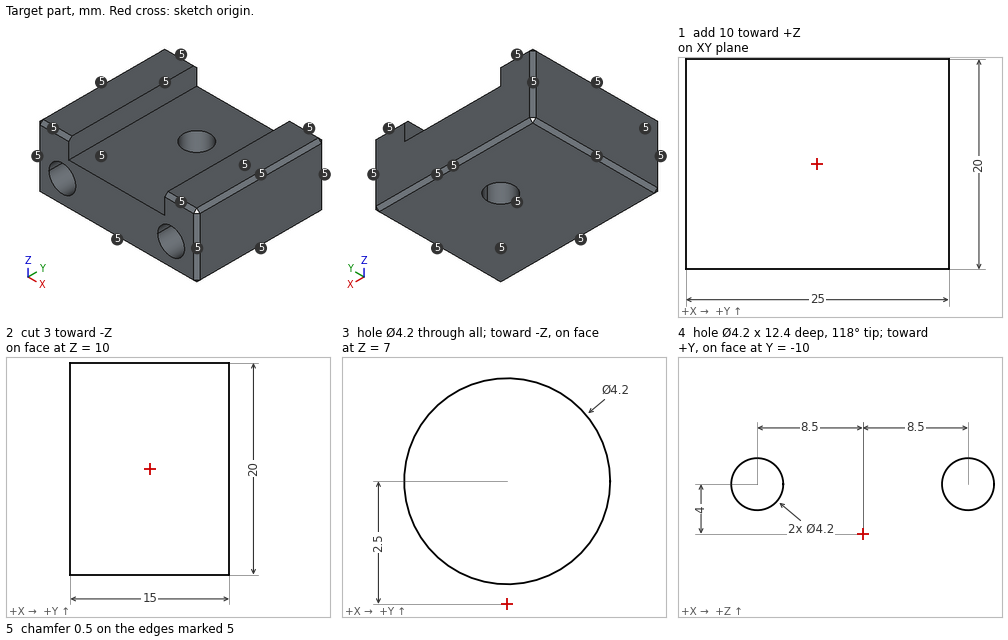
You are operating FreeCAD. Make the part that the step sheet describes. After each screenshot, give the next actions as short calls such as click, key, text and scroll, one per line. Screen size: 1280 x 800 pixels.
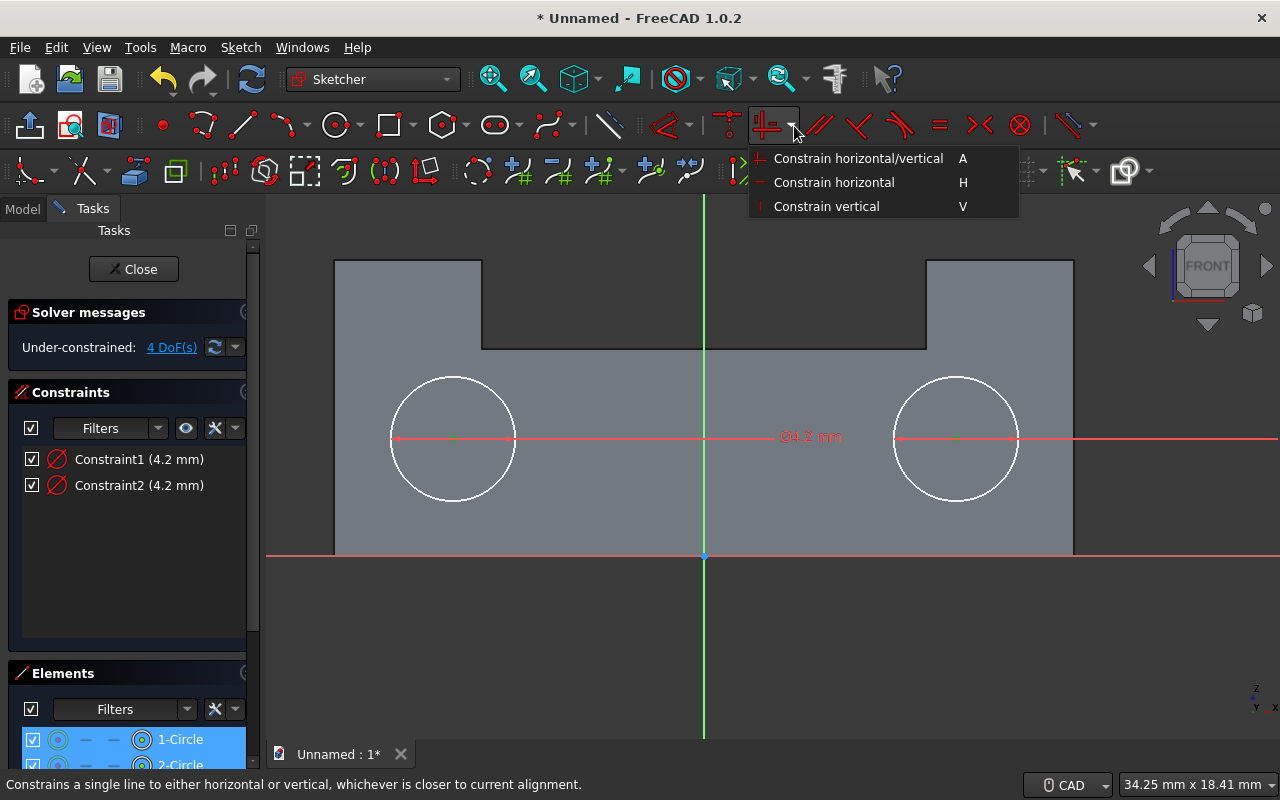
click(884, 182)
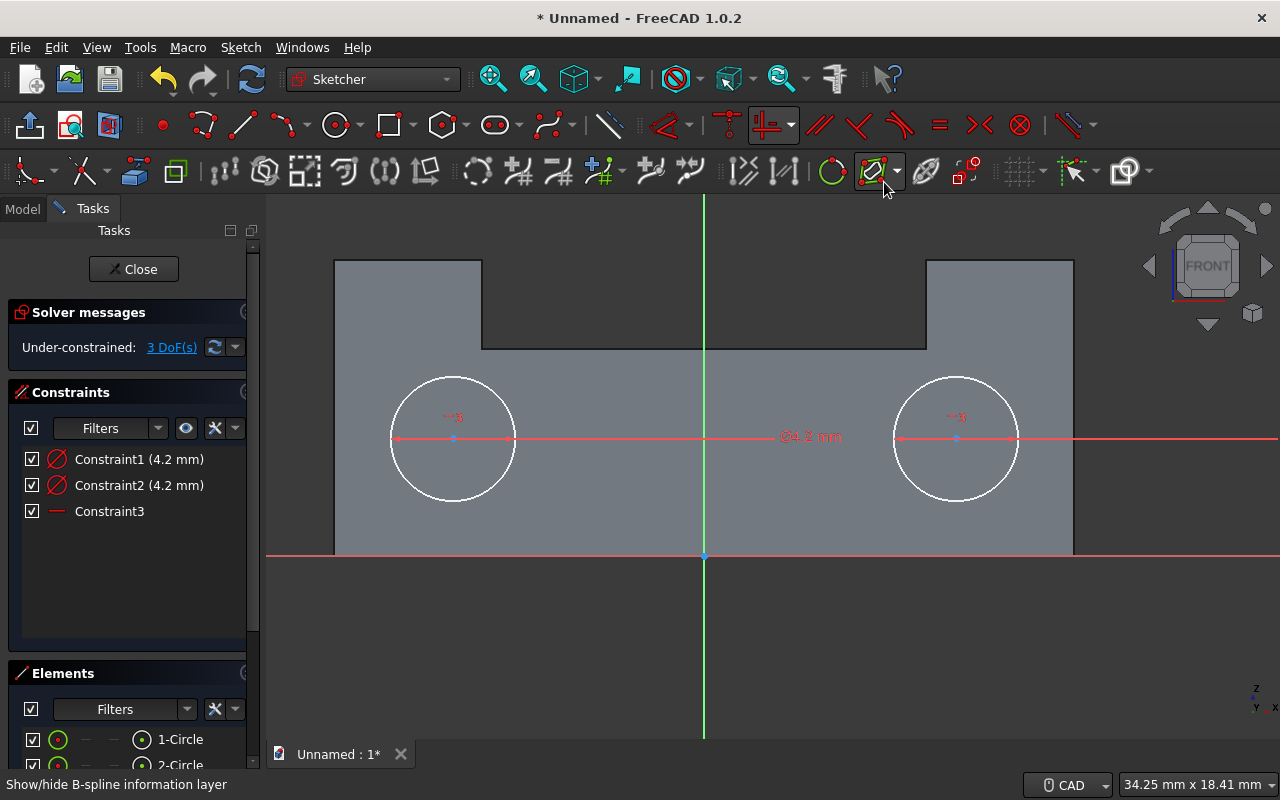
click(664, 126)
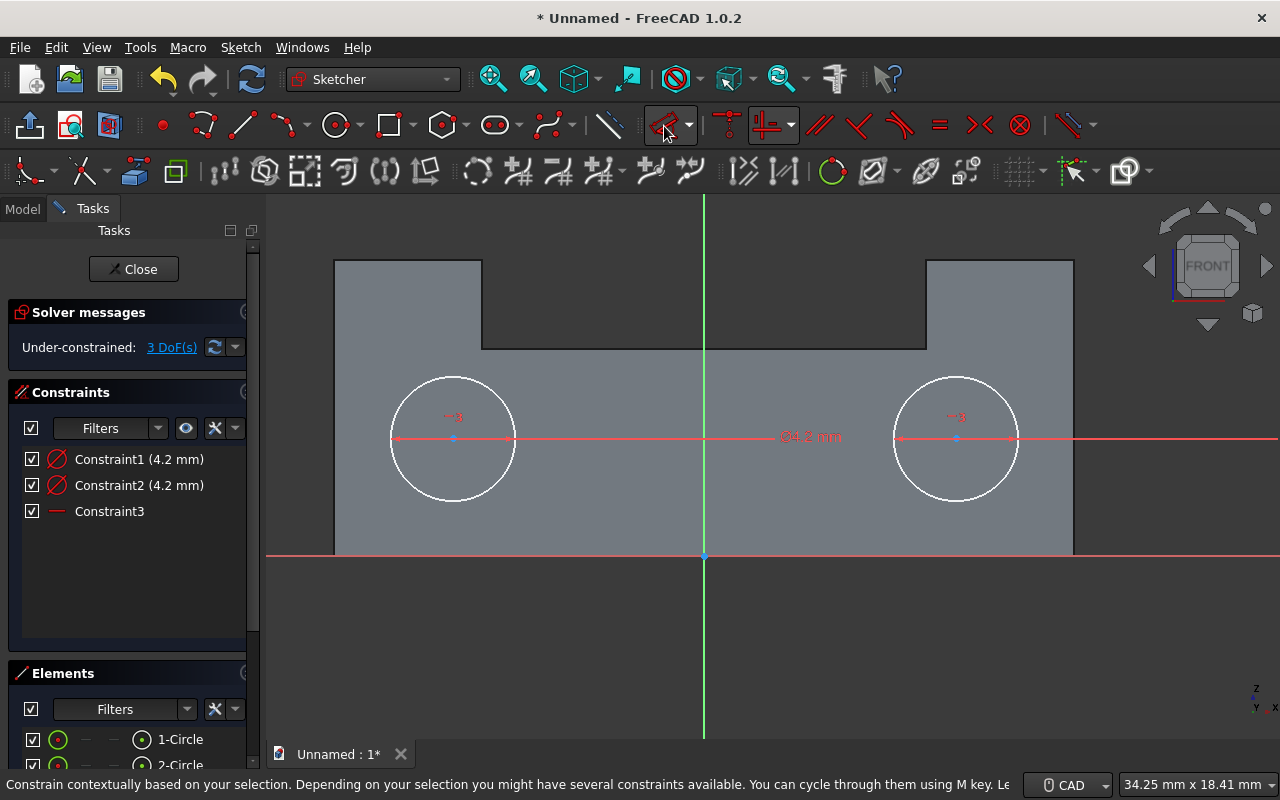
click(453, 439)
click(419, 471)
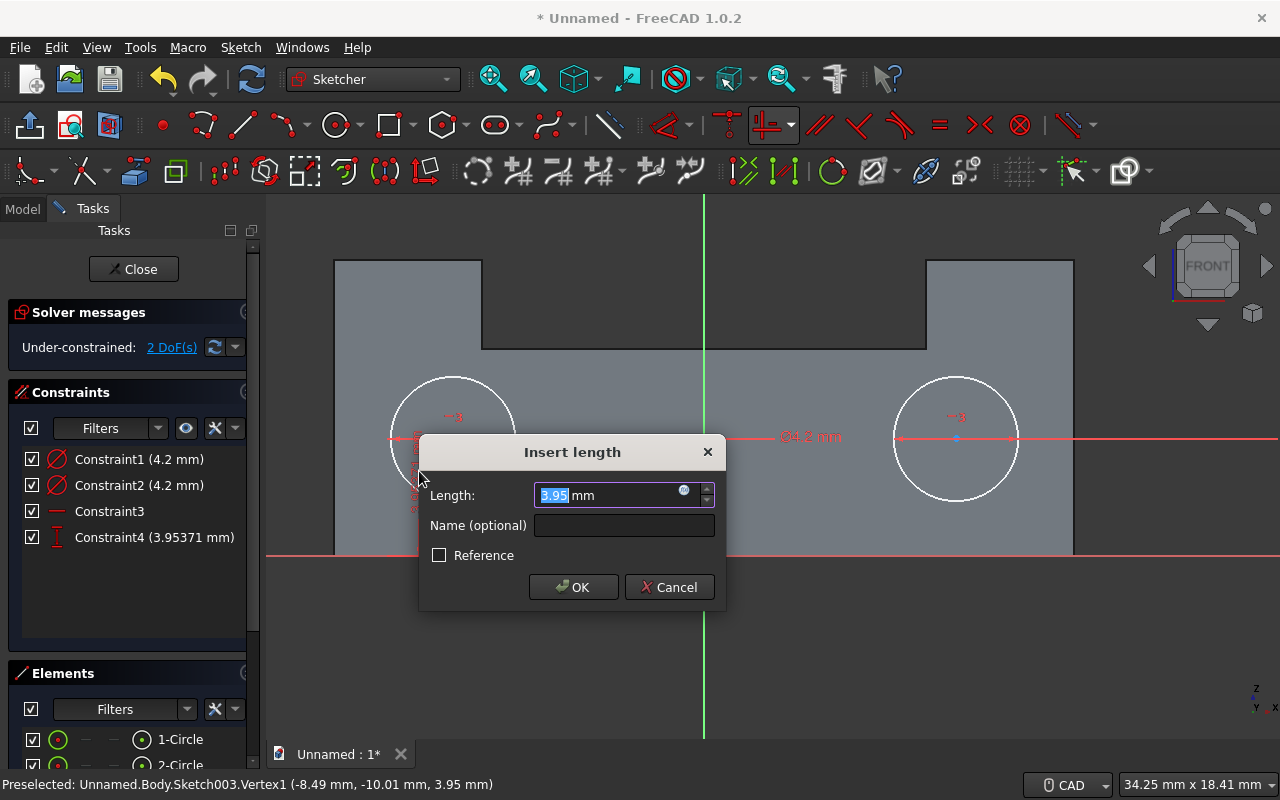
text(4)
key(Return)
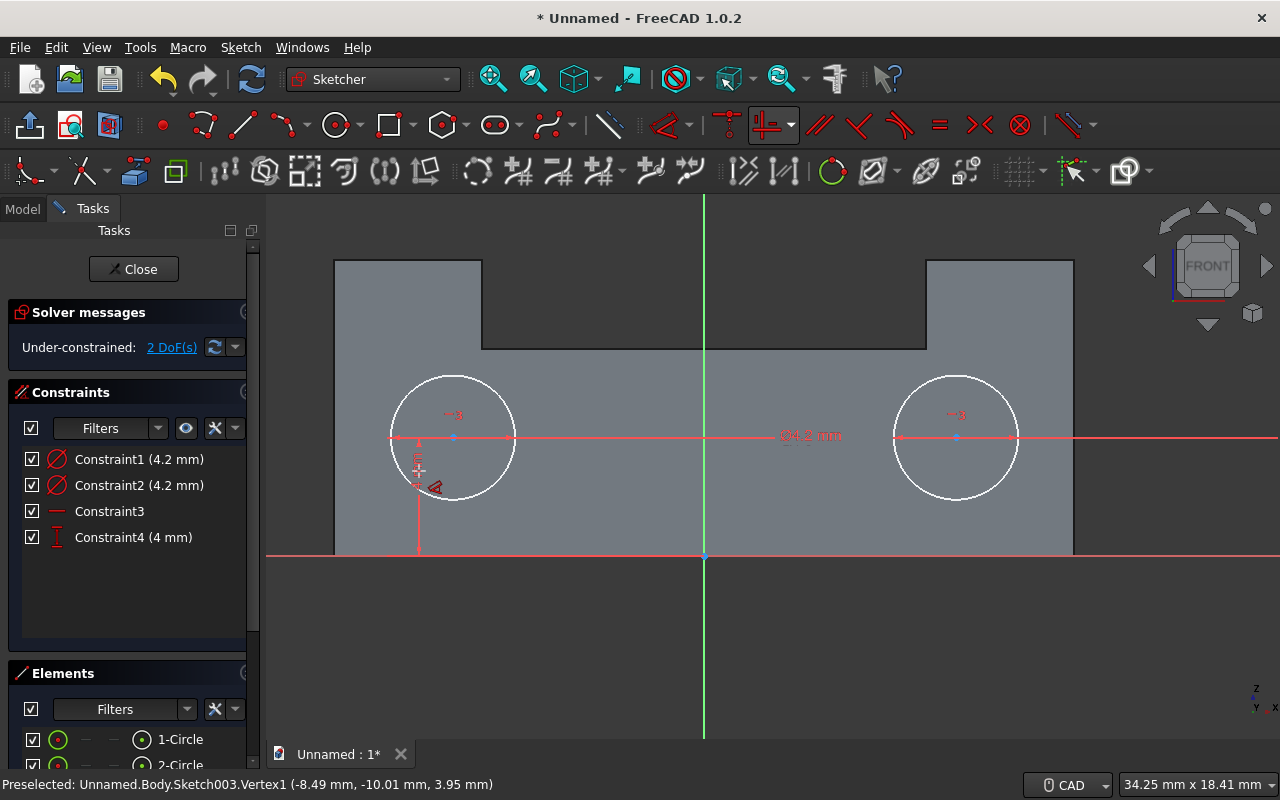
click(453, 438)
click(579, 590)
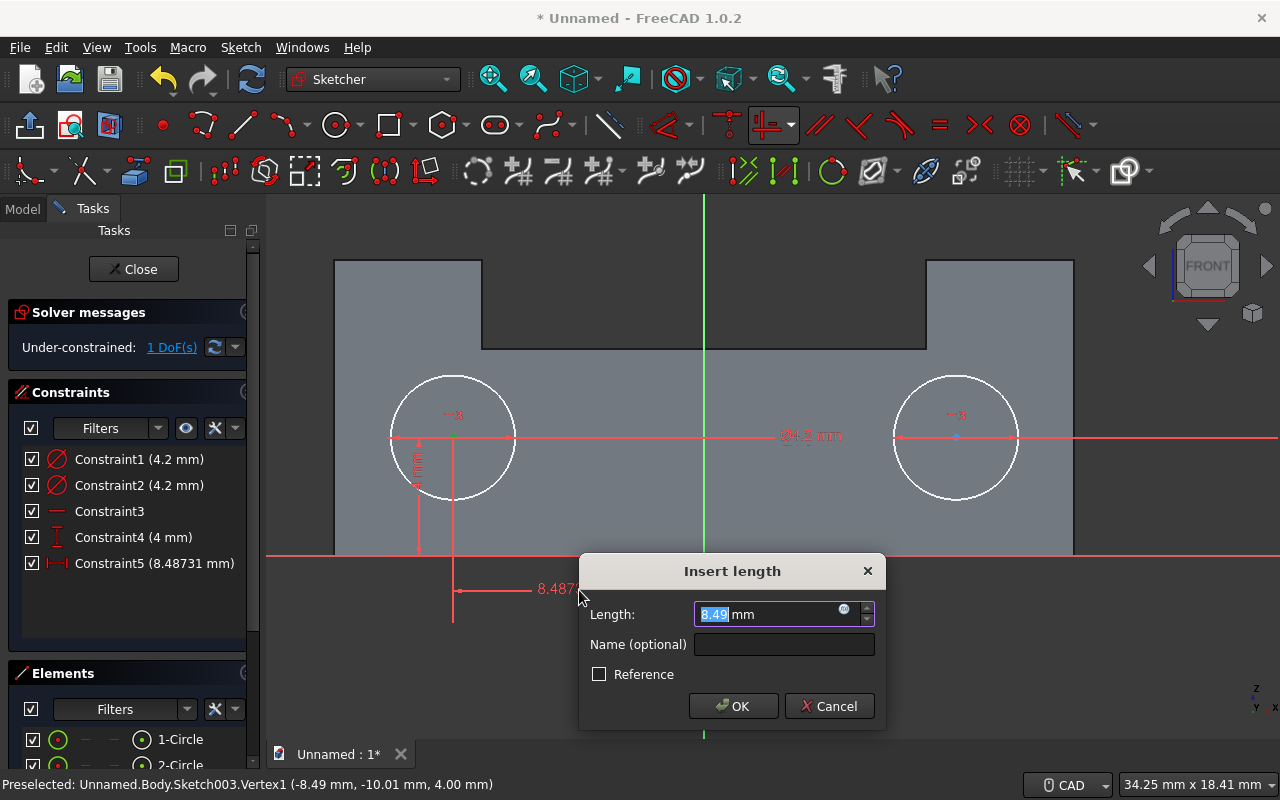
text(8.5)
key(Return)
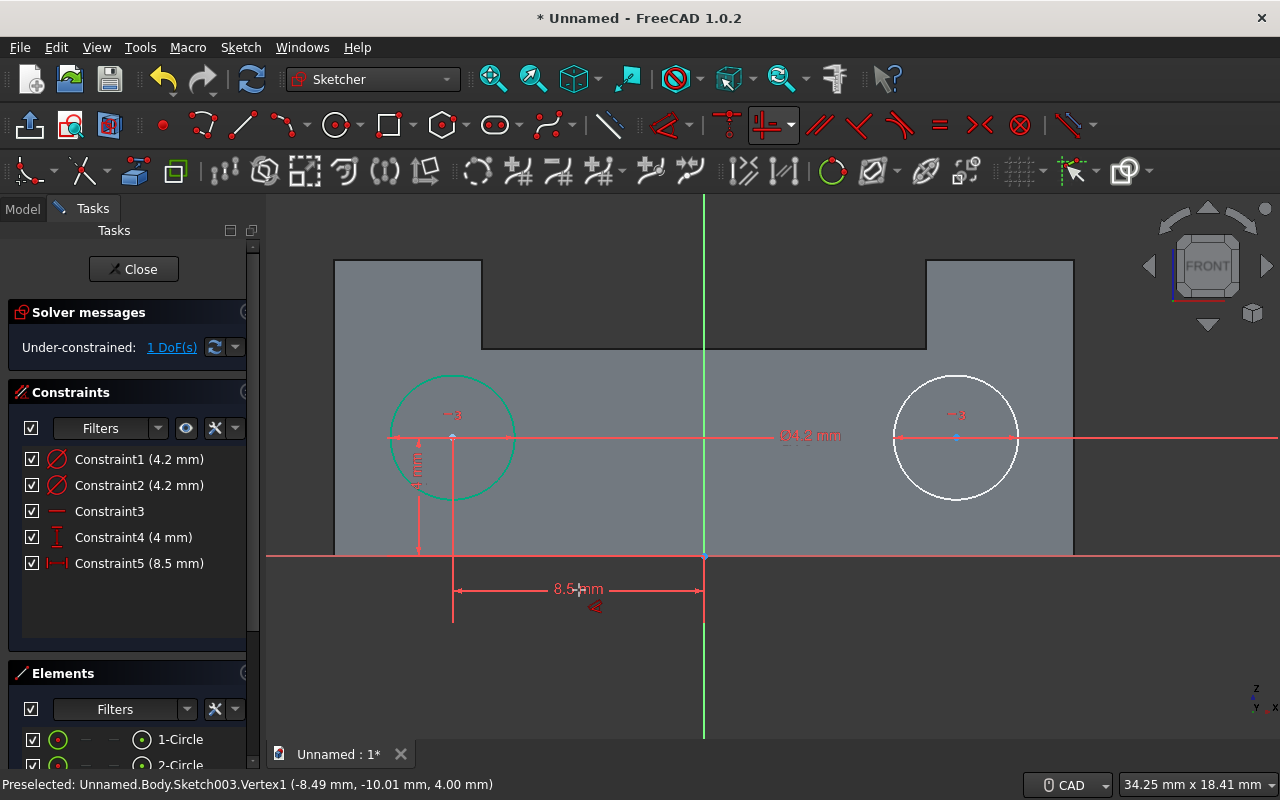
click(956, 438)
click(830, 590)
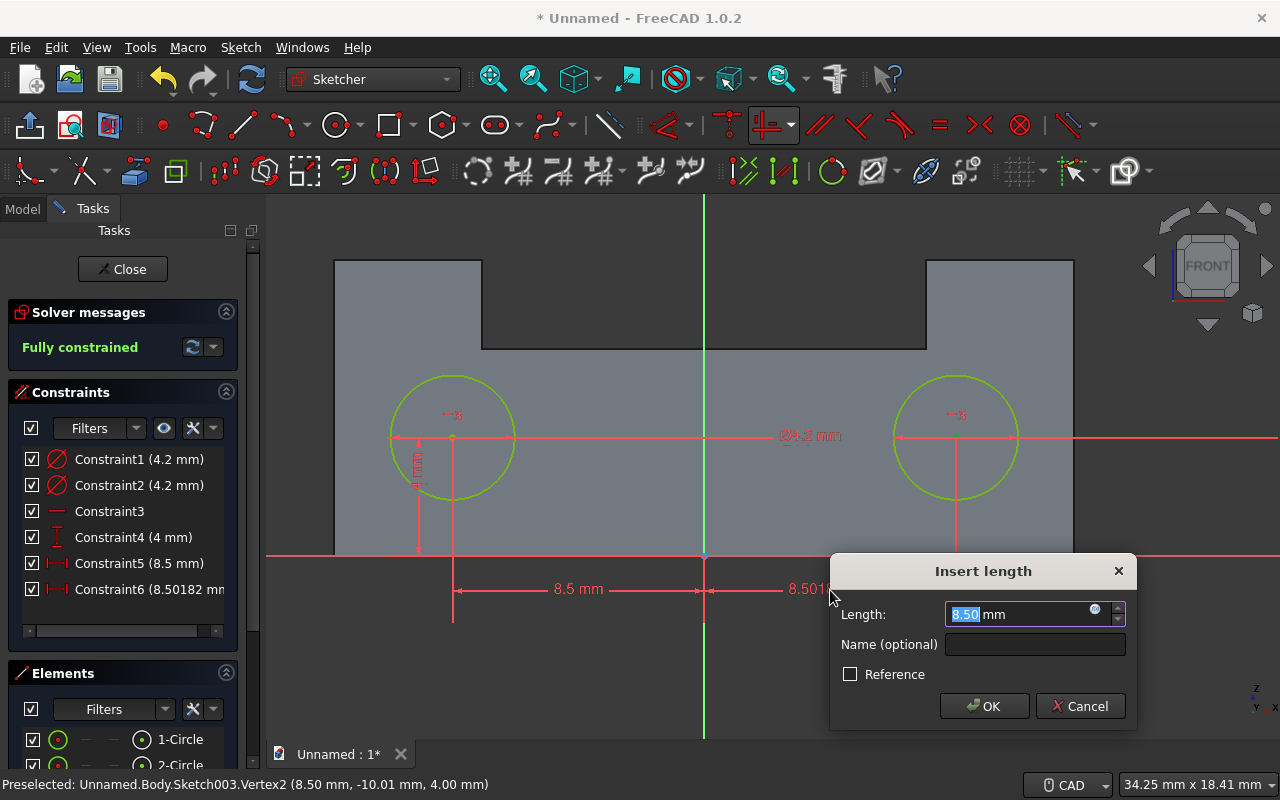
text(8.5)
key(Return)
key(Escape)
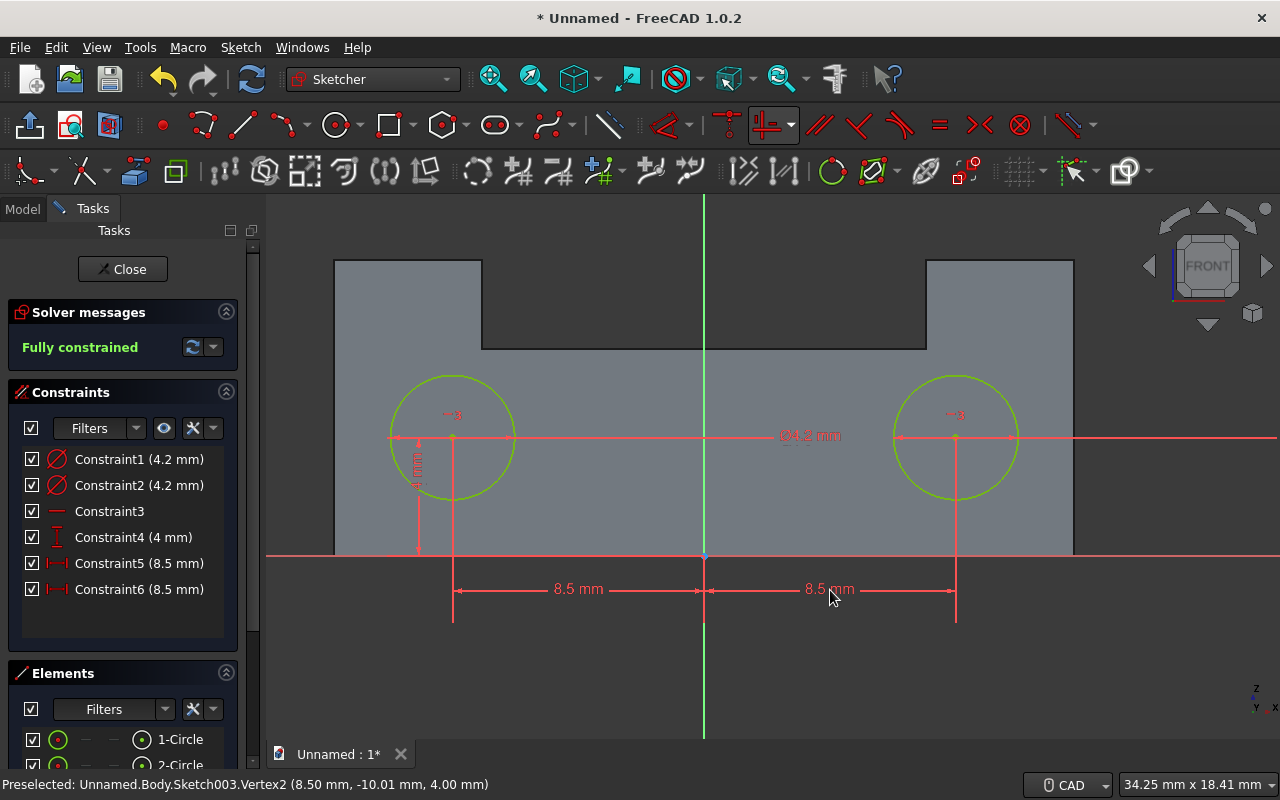
click(123, 269)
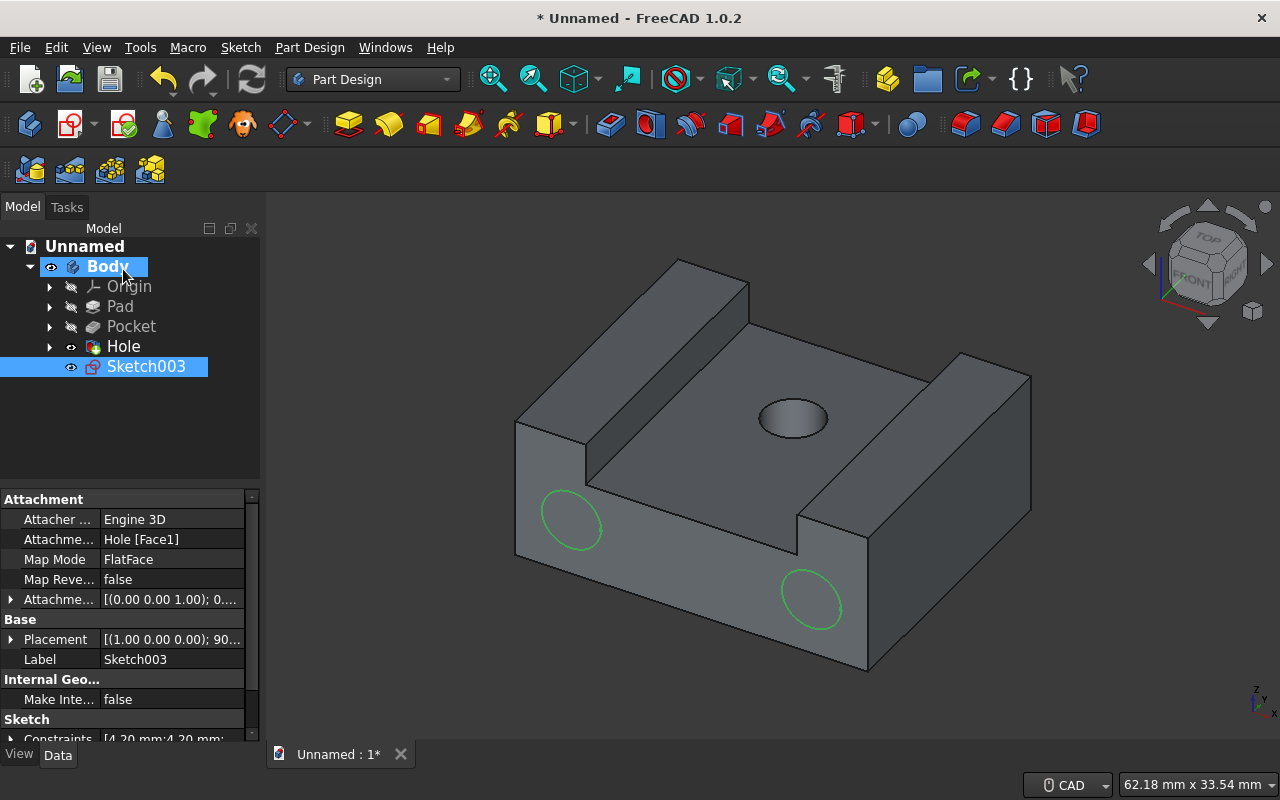
click(652, 124)